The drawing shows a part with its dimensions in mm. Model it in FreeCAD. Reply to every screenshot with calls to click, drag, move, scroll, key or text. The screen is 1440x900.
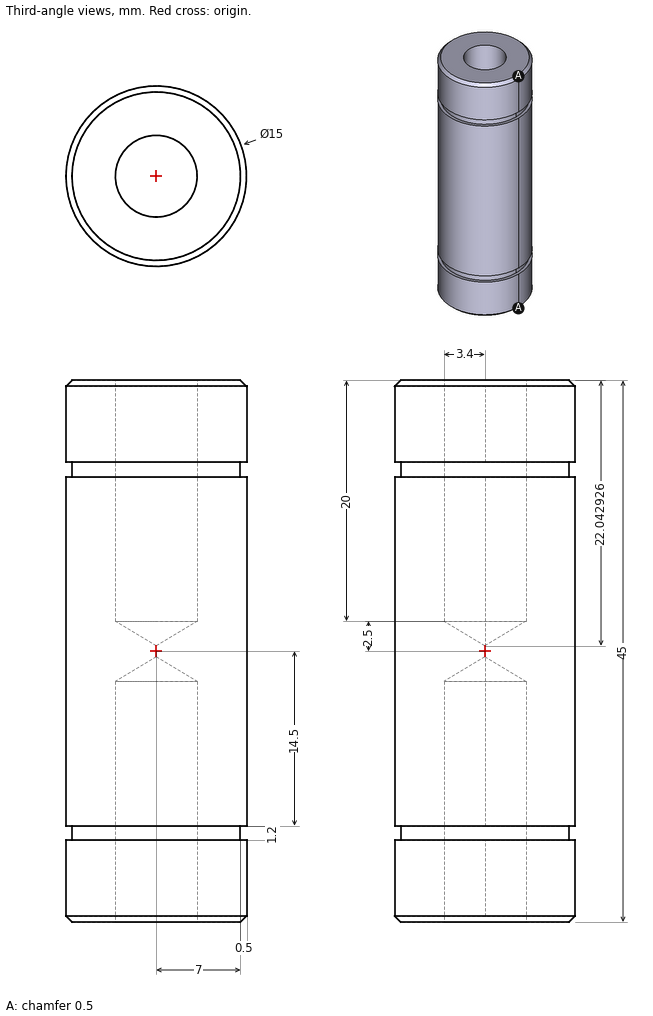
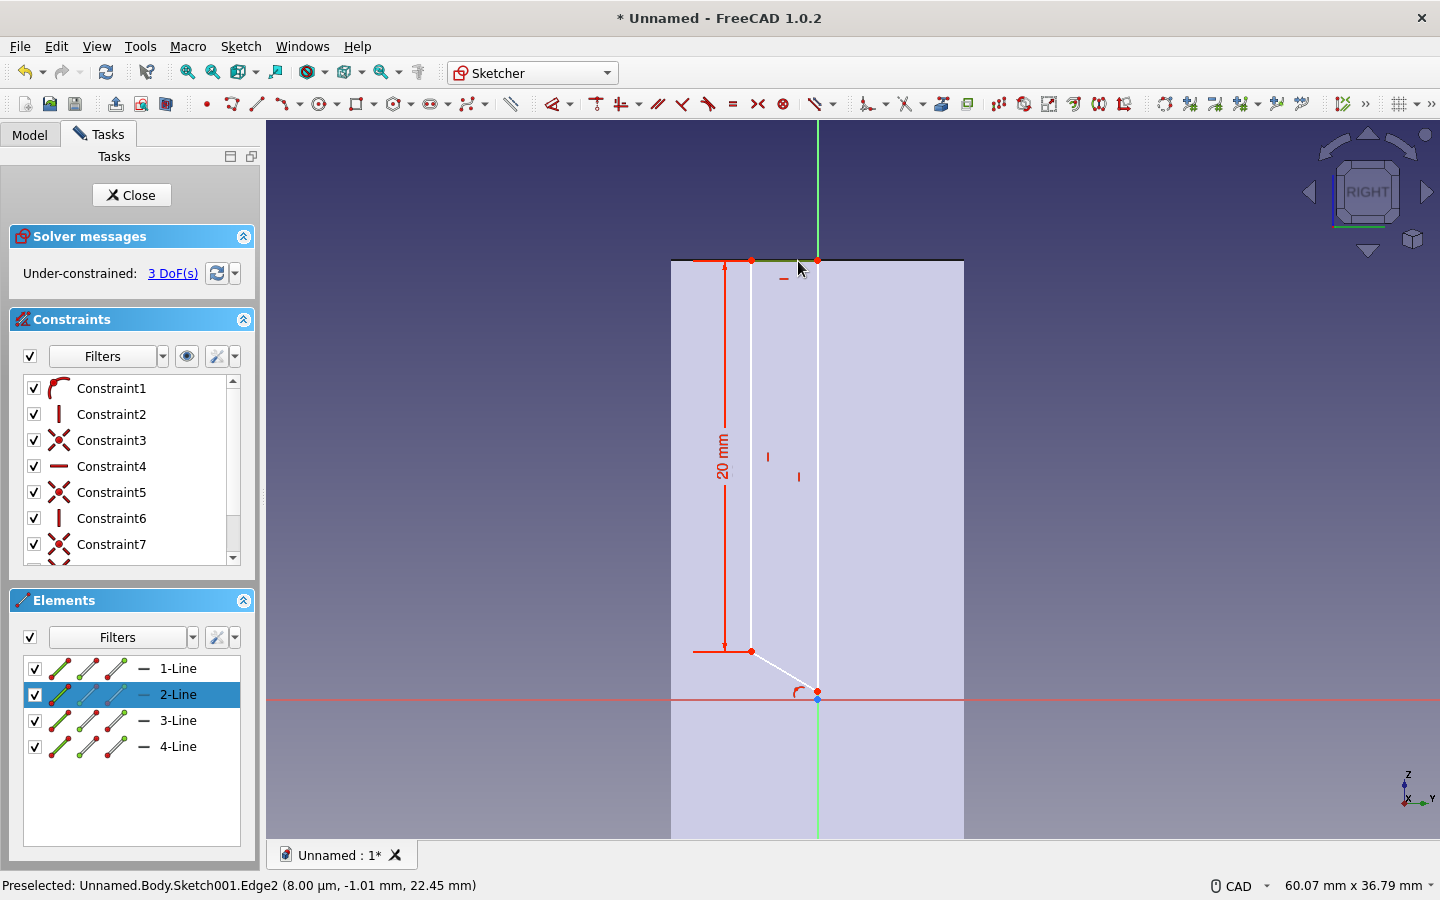
click(570, 104)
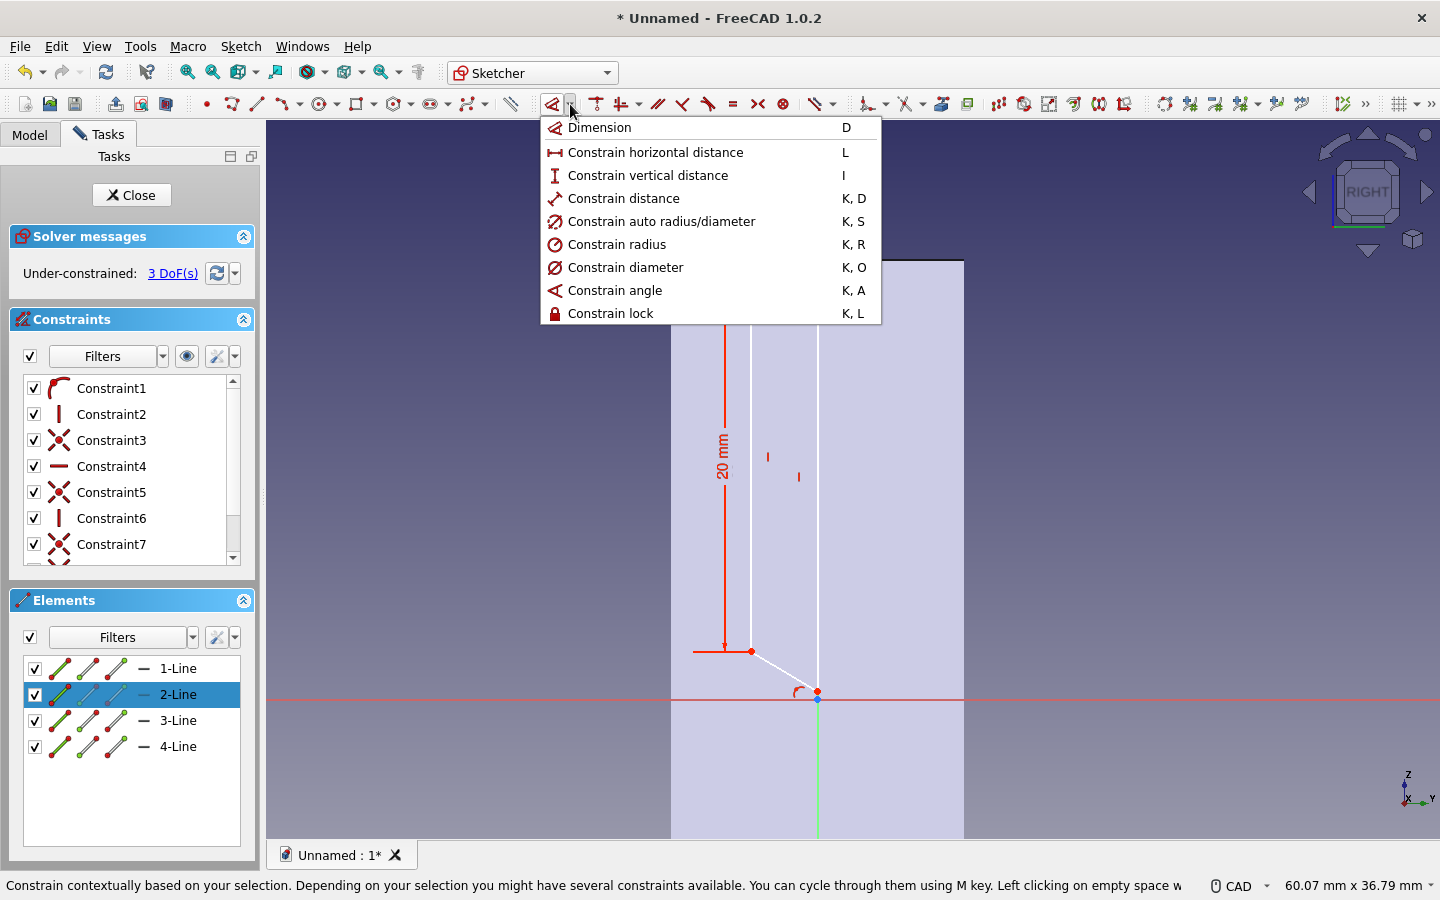
click(711, 152)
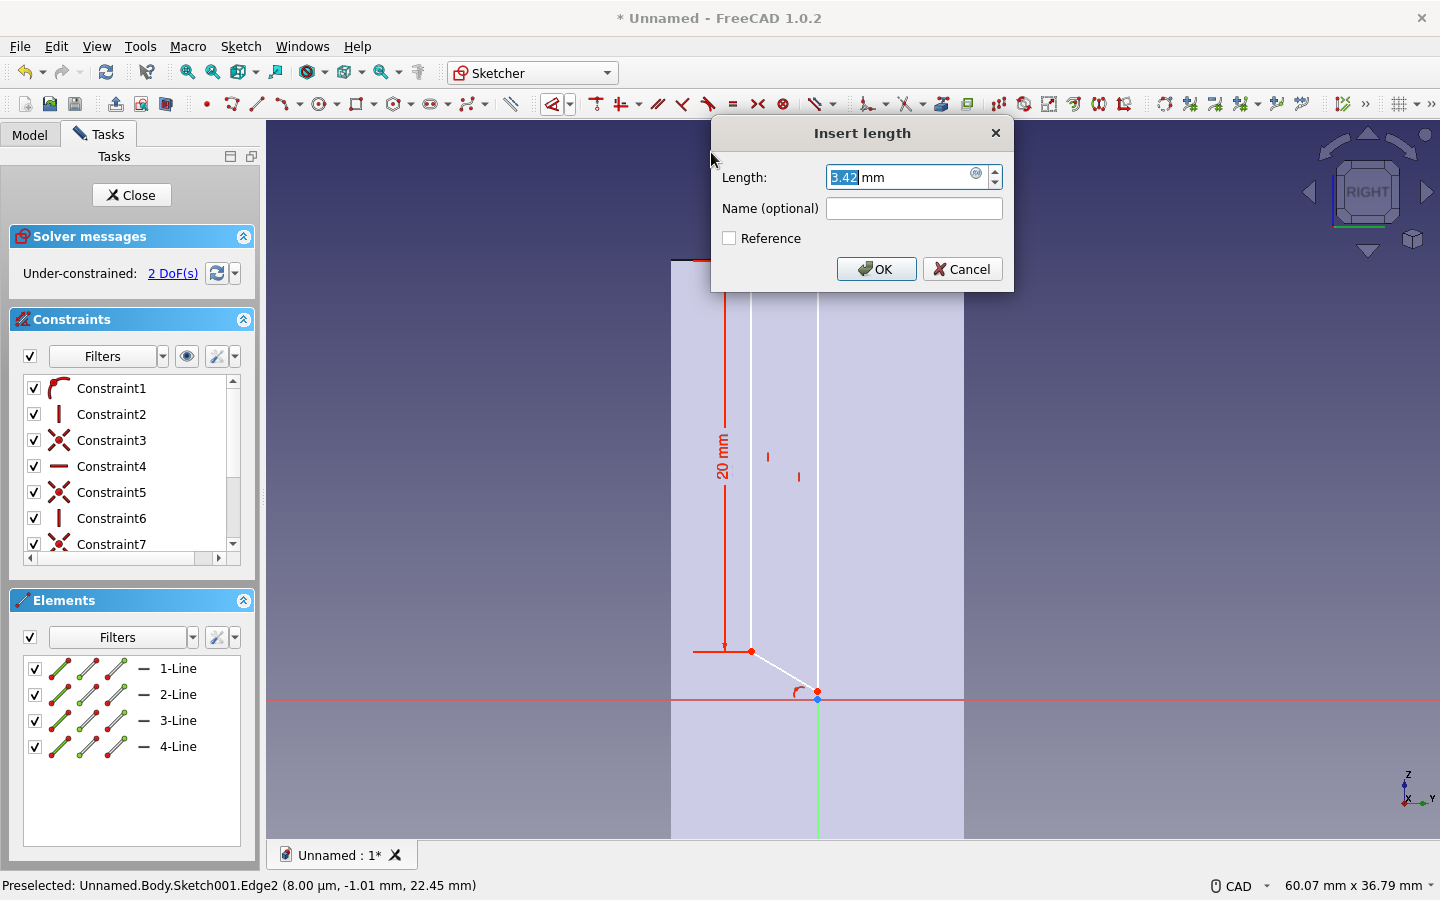
text(3.4)
key(Return)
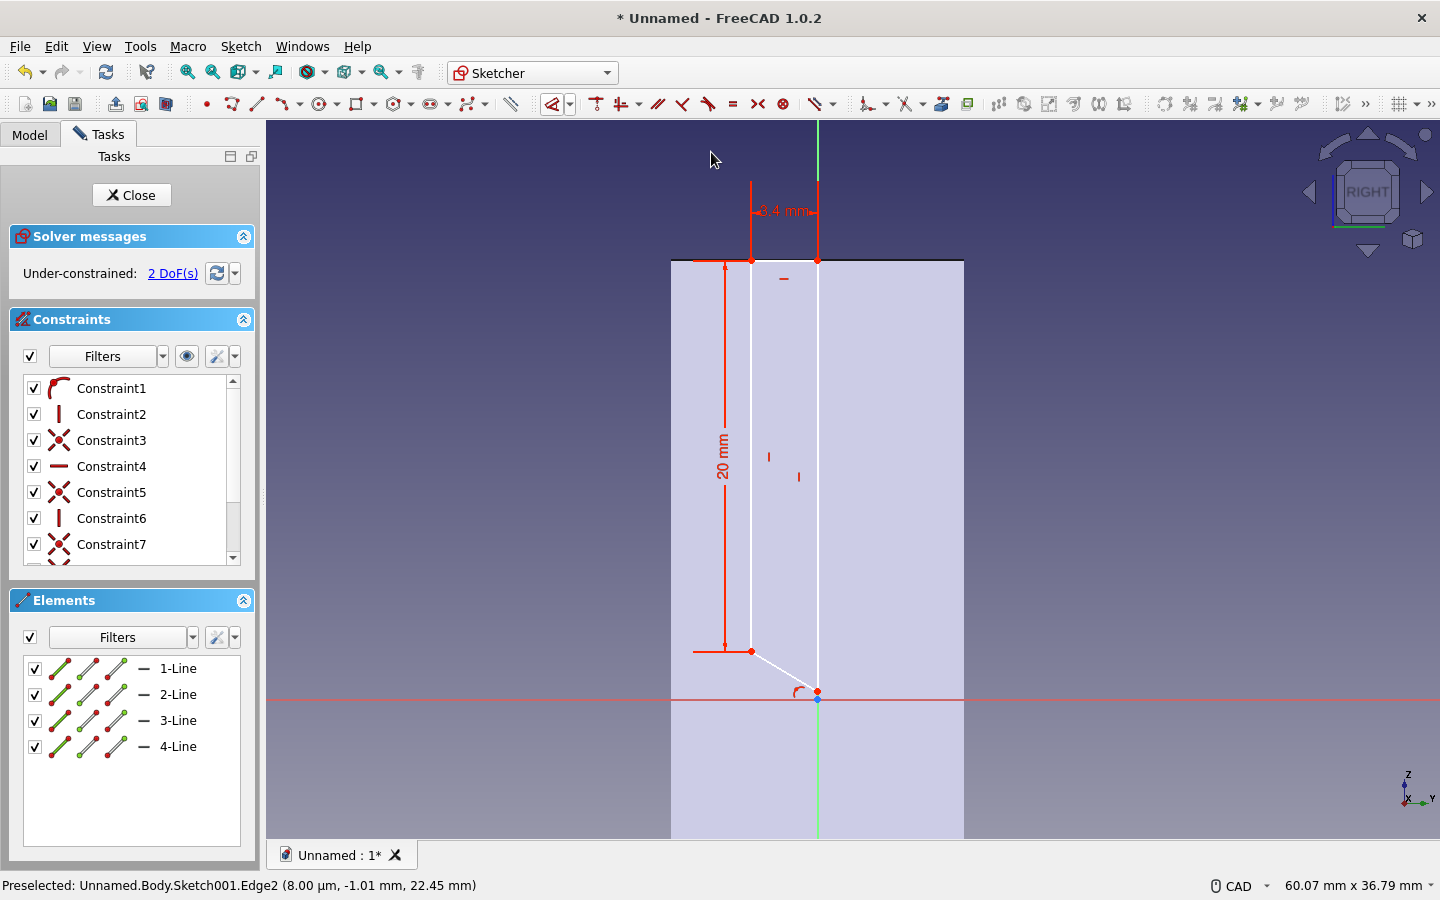
click(751, 652)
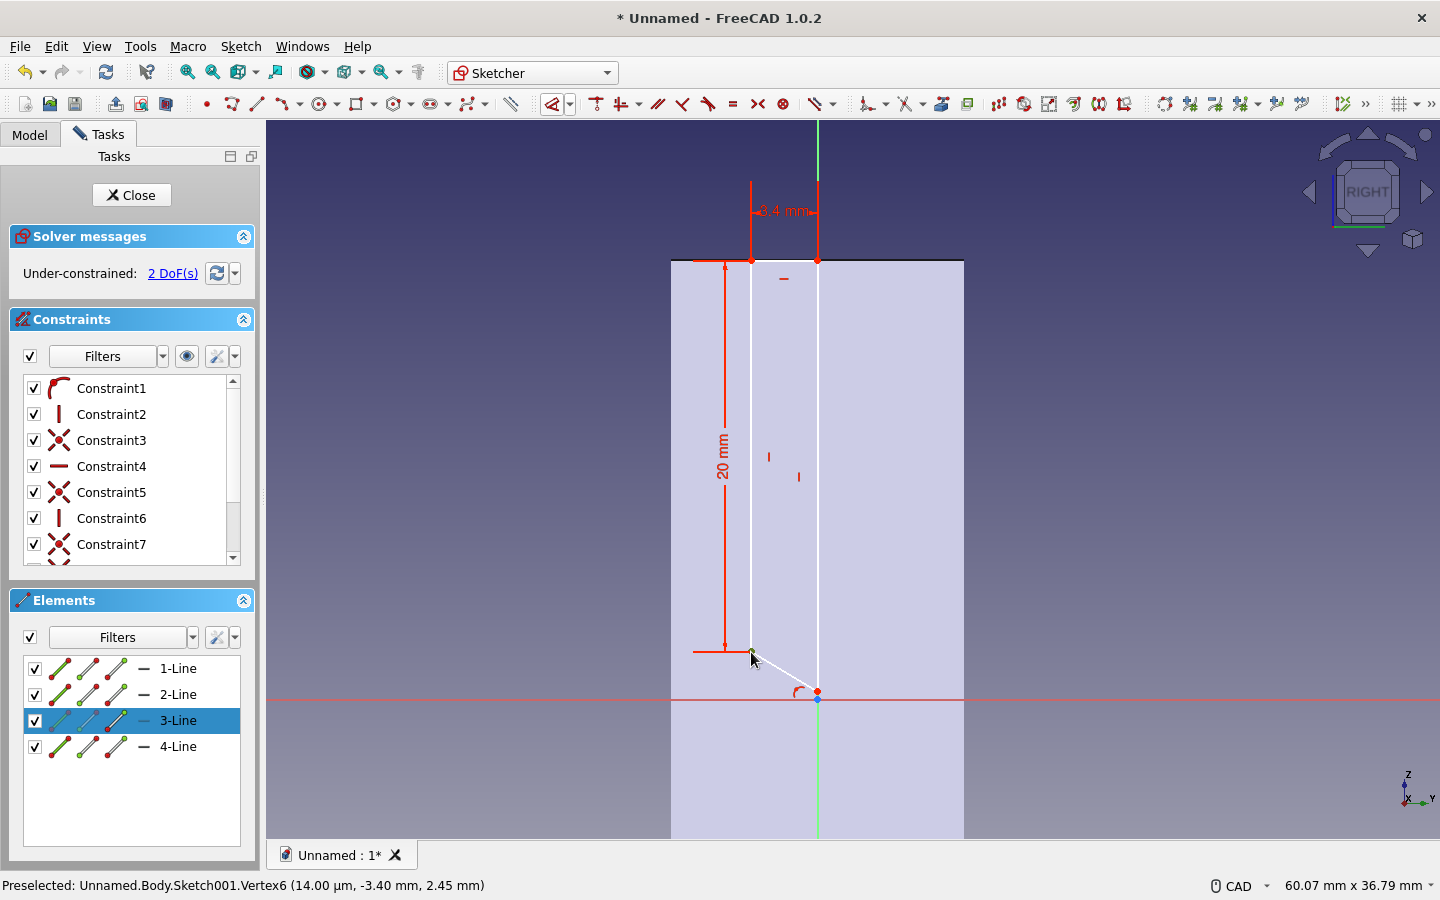
click(570, 104)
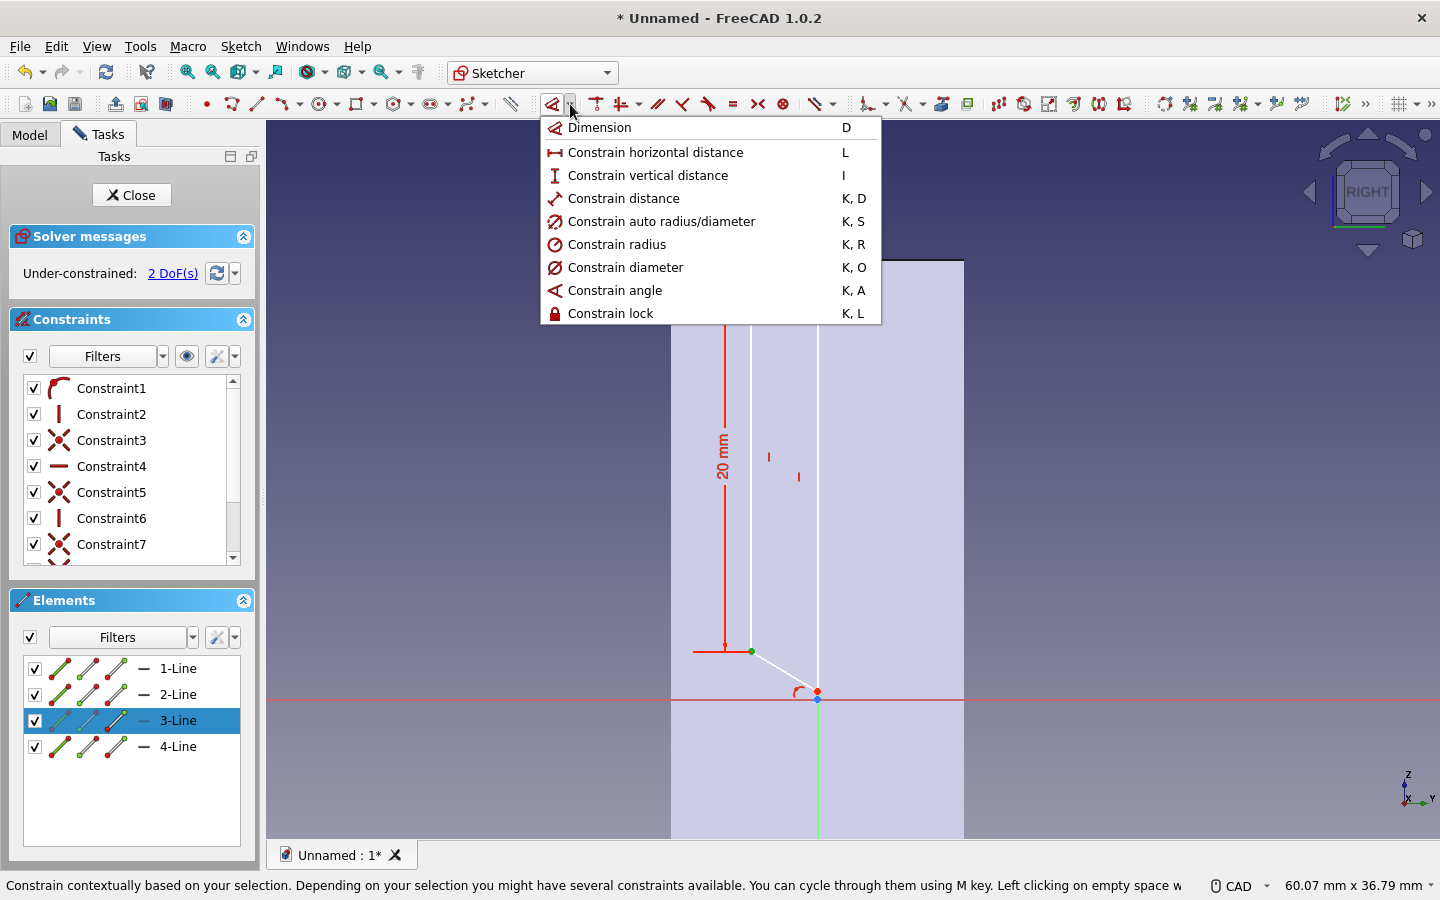
click(711, 176)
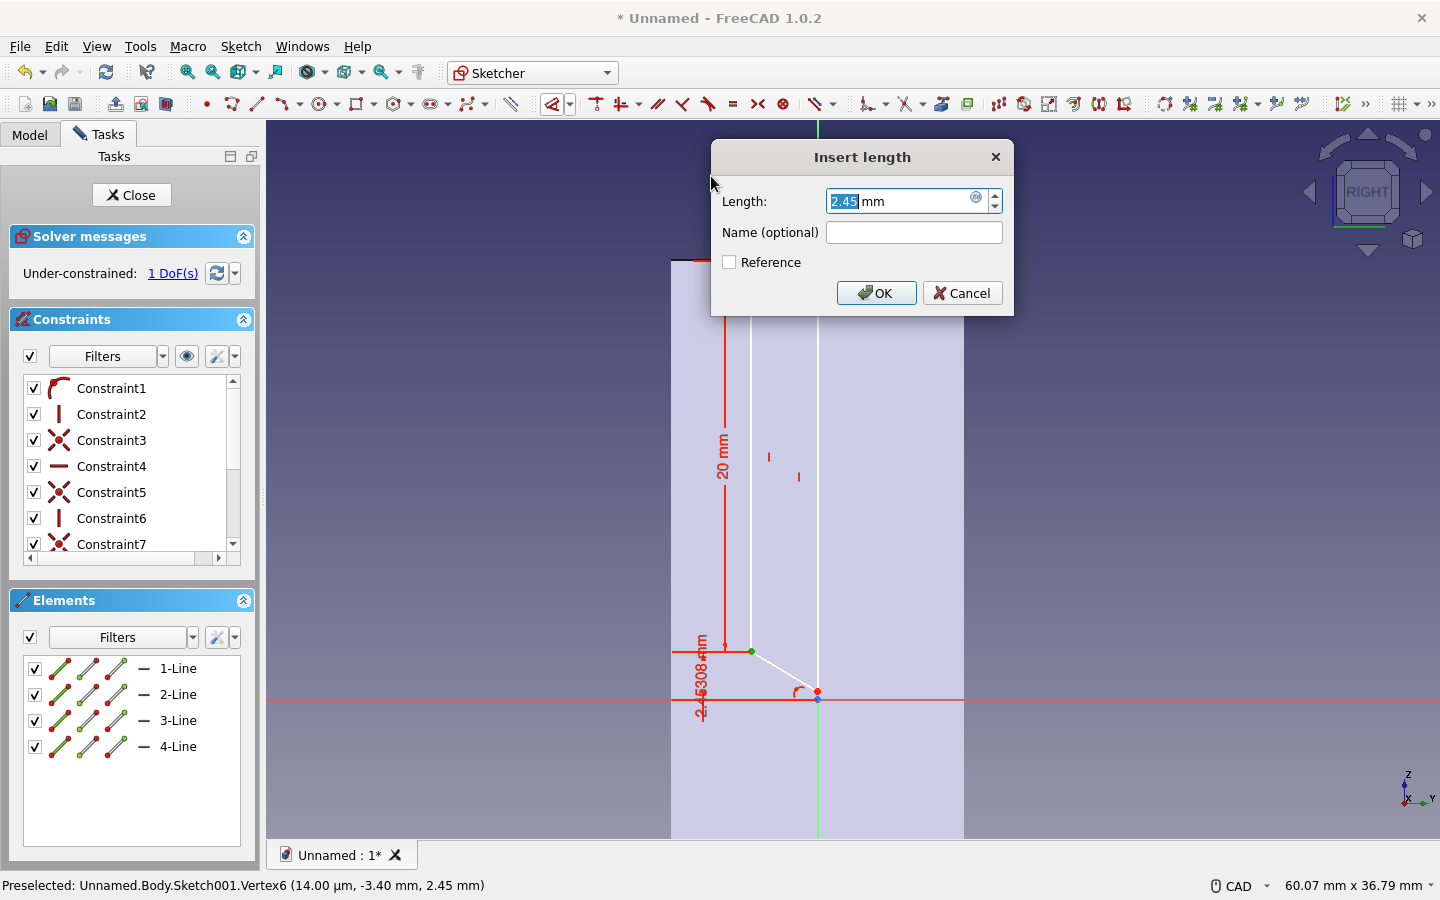
text(2.5)
key(Return)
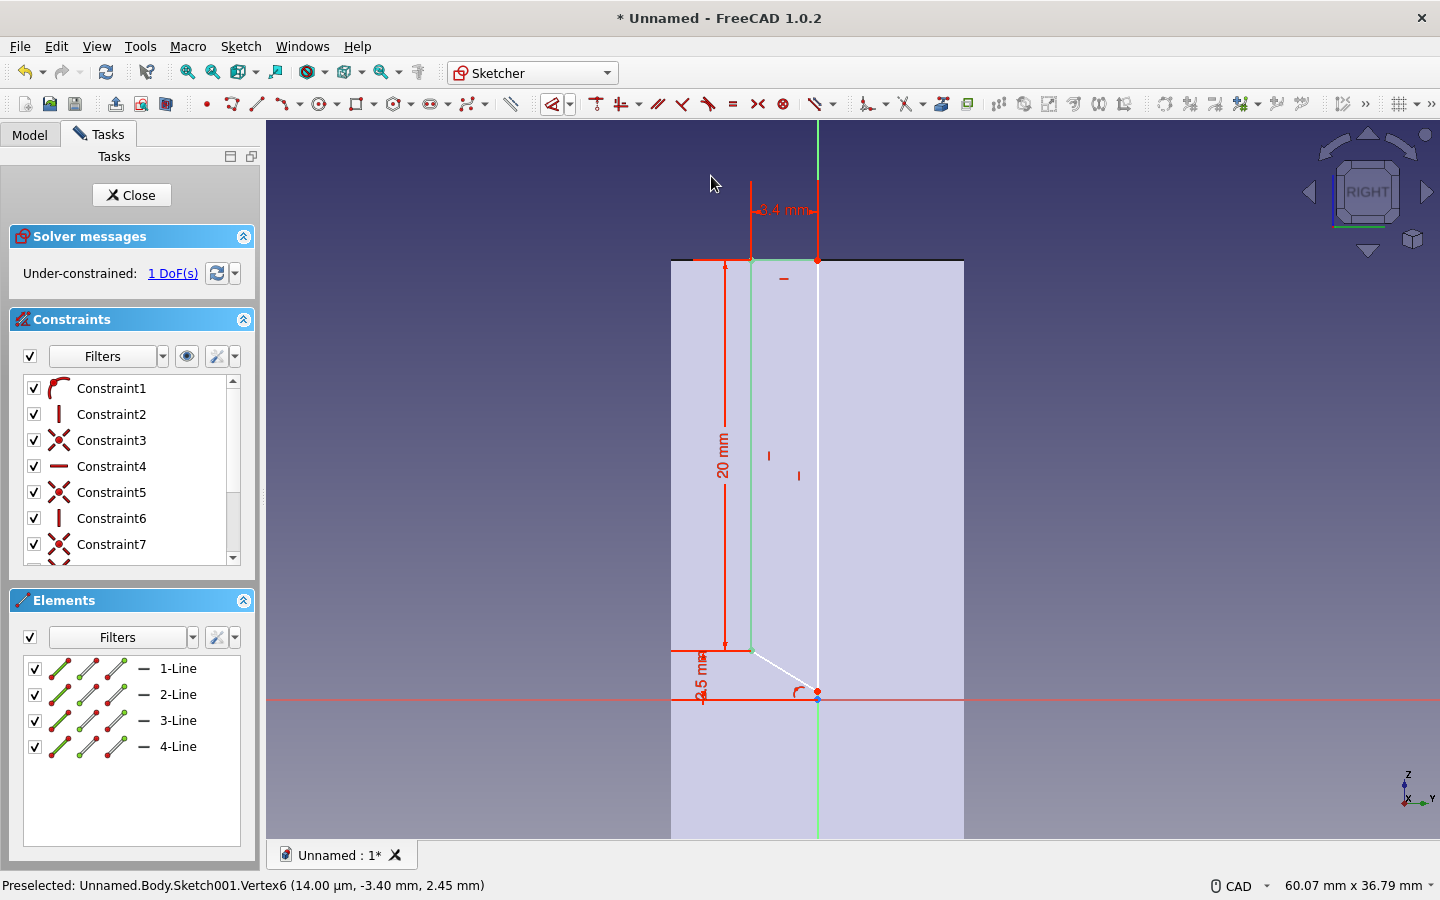
click(818, 562)